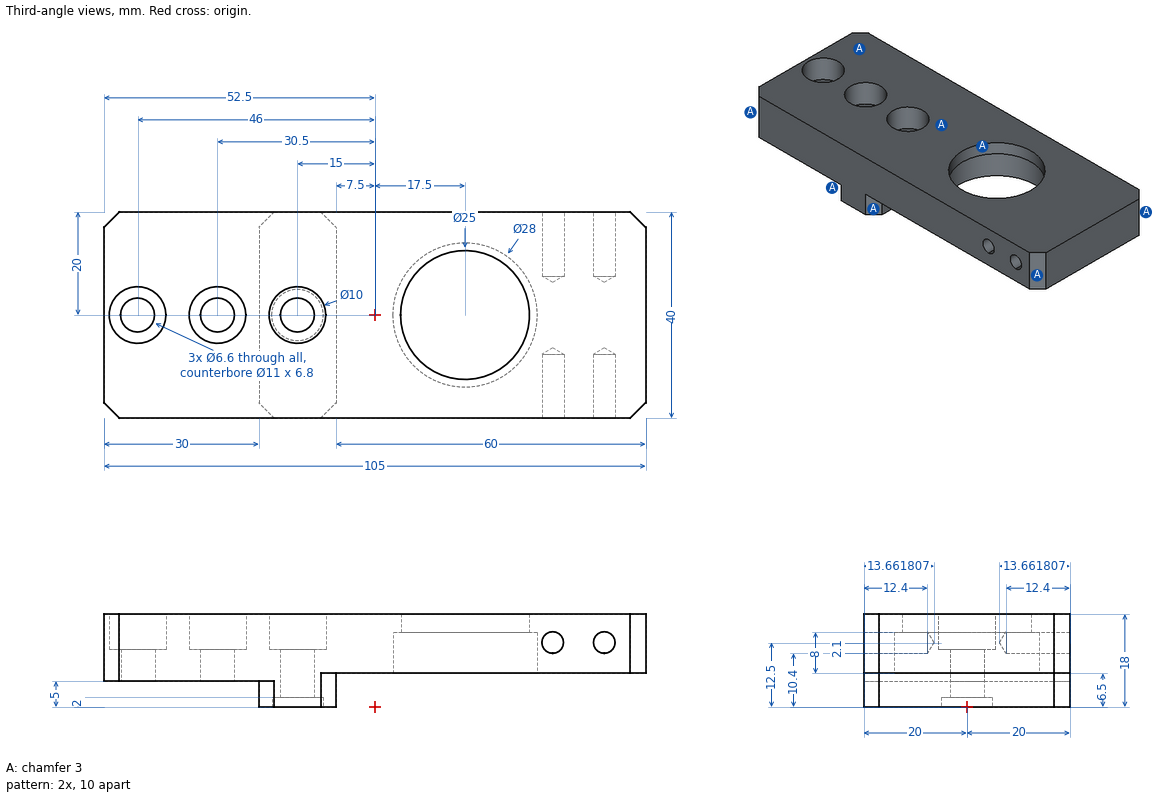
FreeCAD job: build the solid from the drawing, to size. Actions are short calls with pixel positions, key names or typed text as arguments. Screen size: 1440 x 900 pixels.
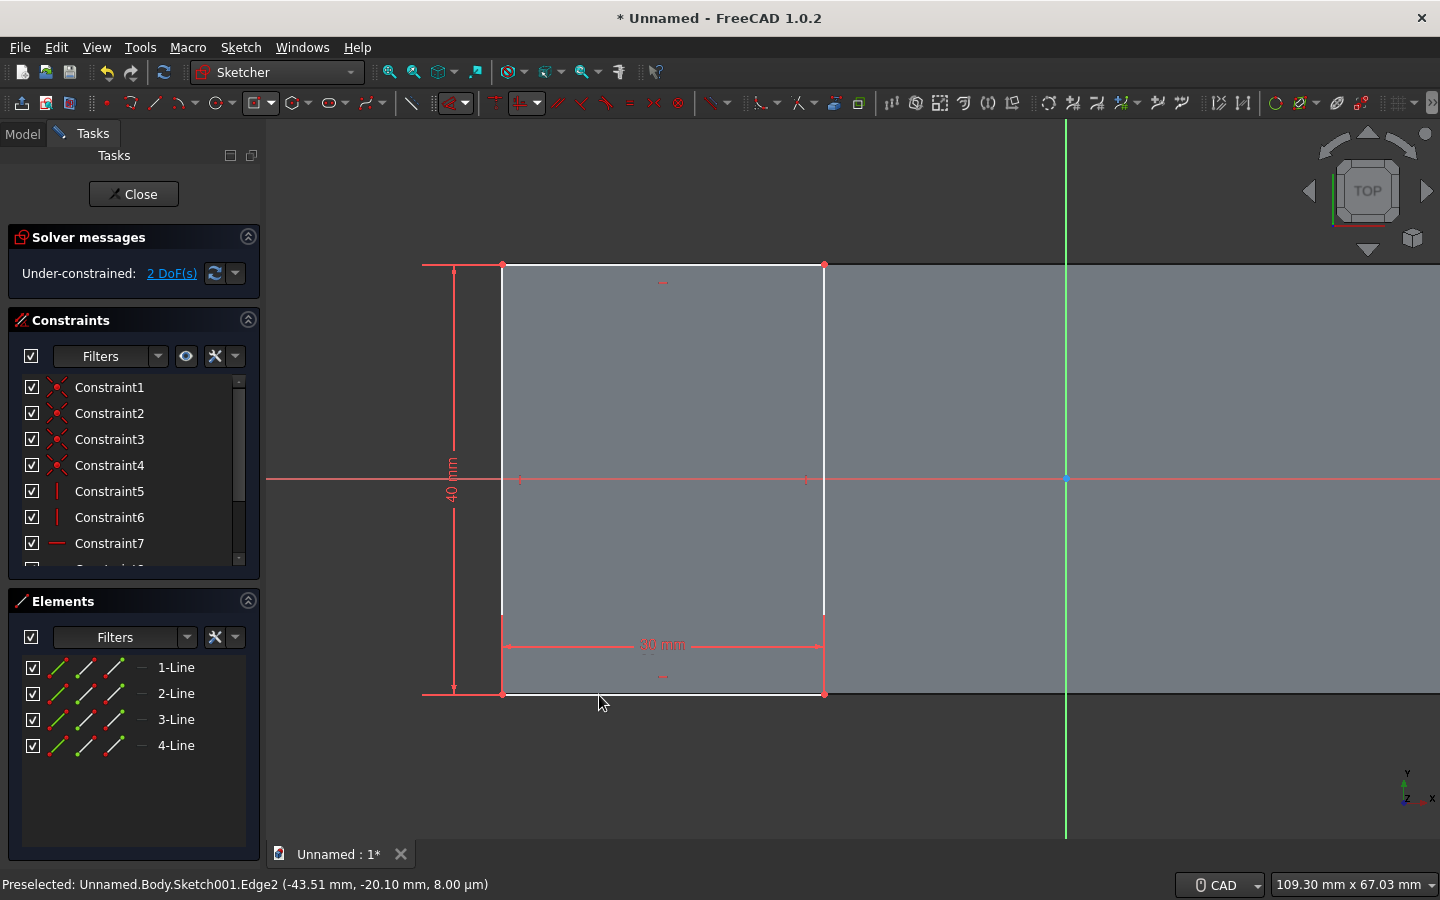
click(502, 265)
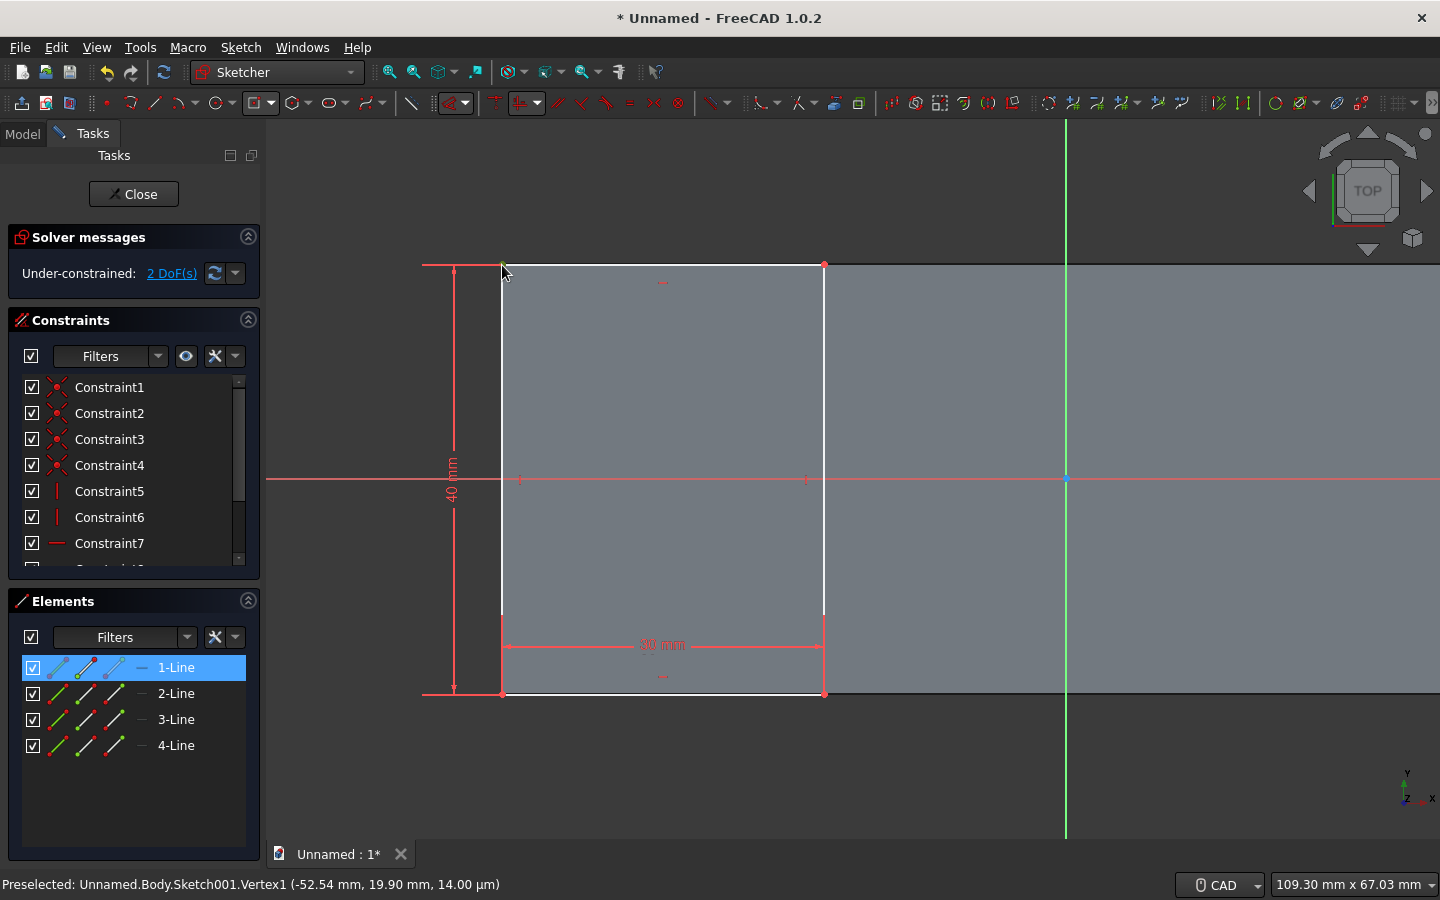
click(468, 104)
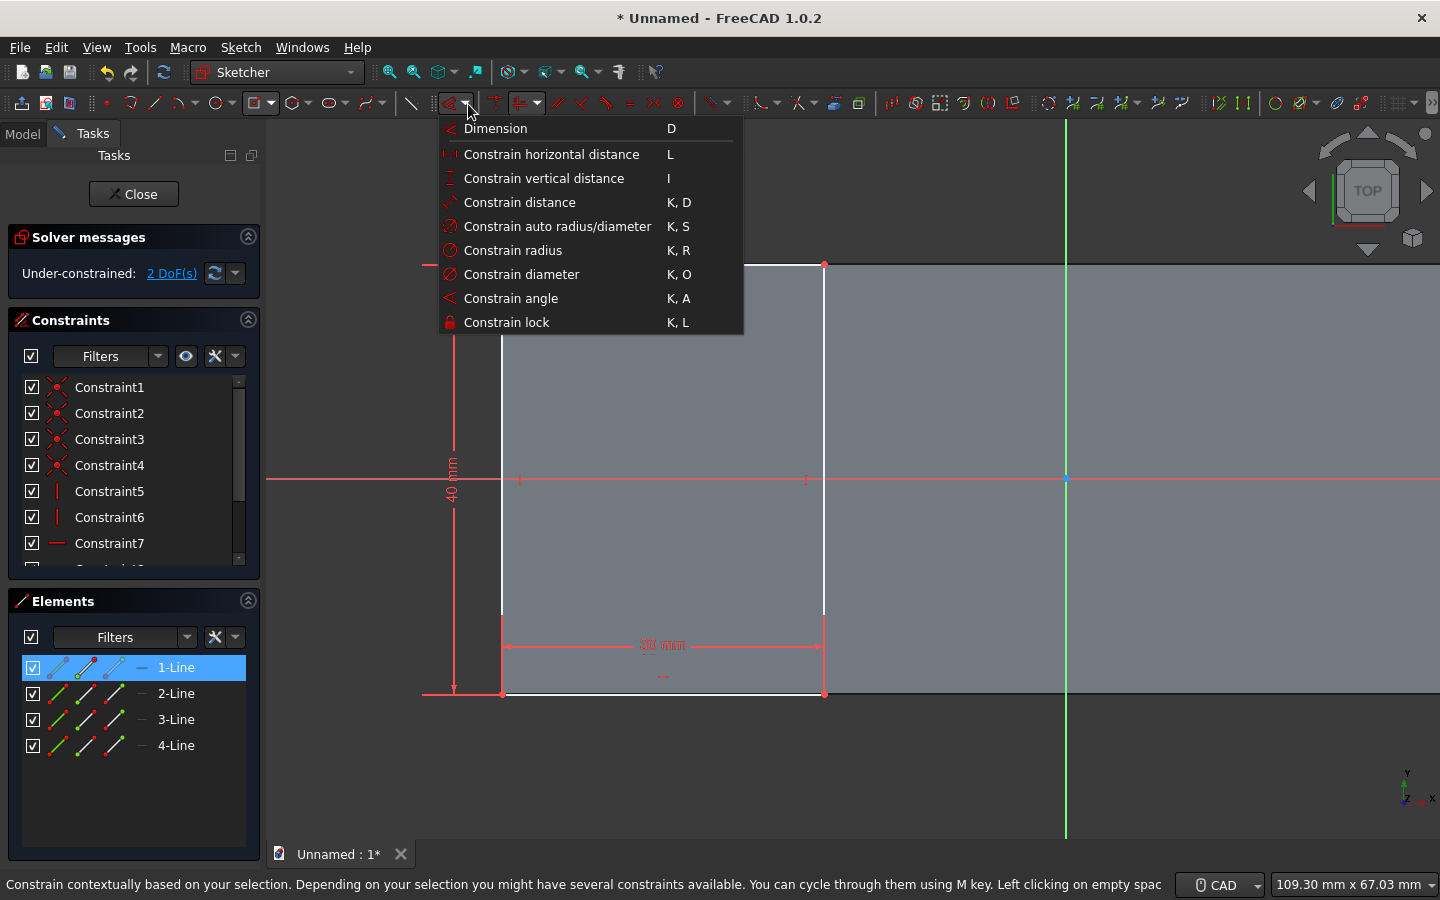
click(591, 178)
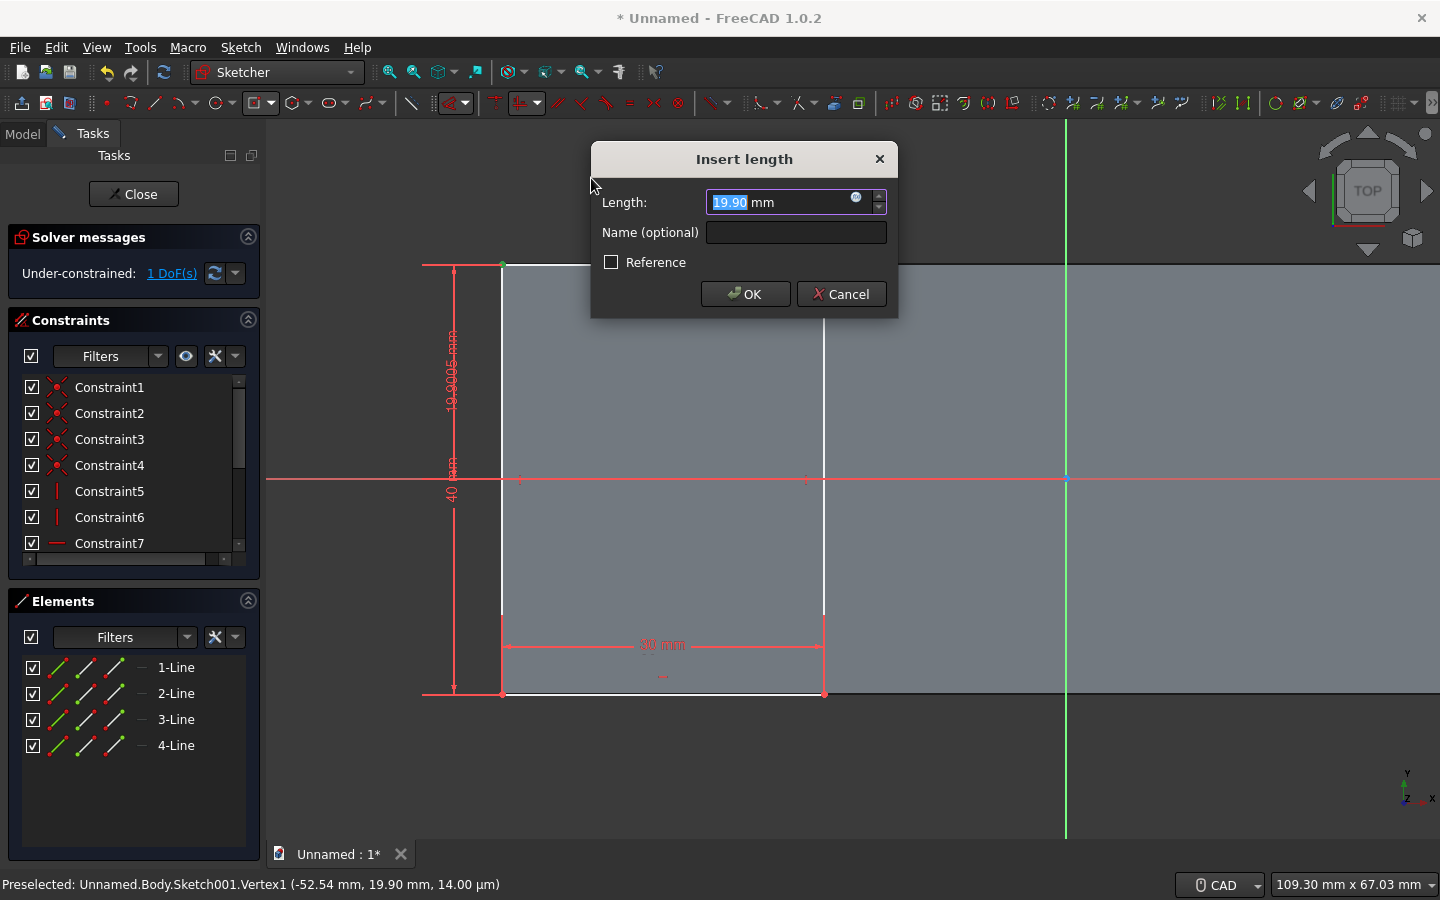
text(20)
key(Return)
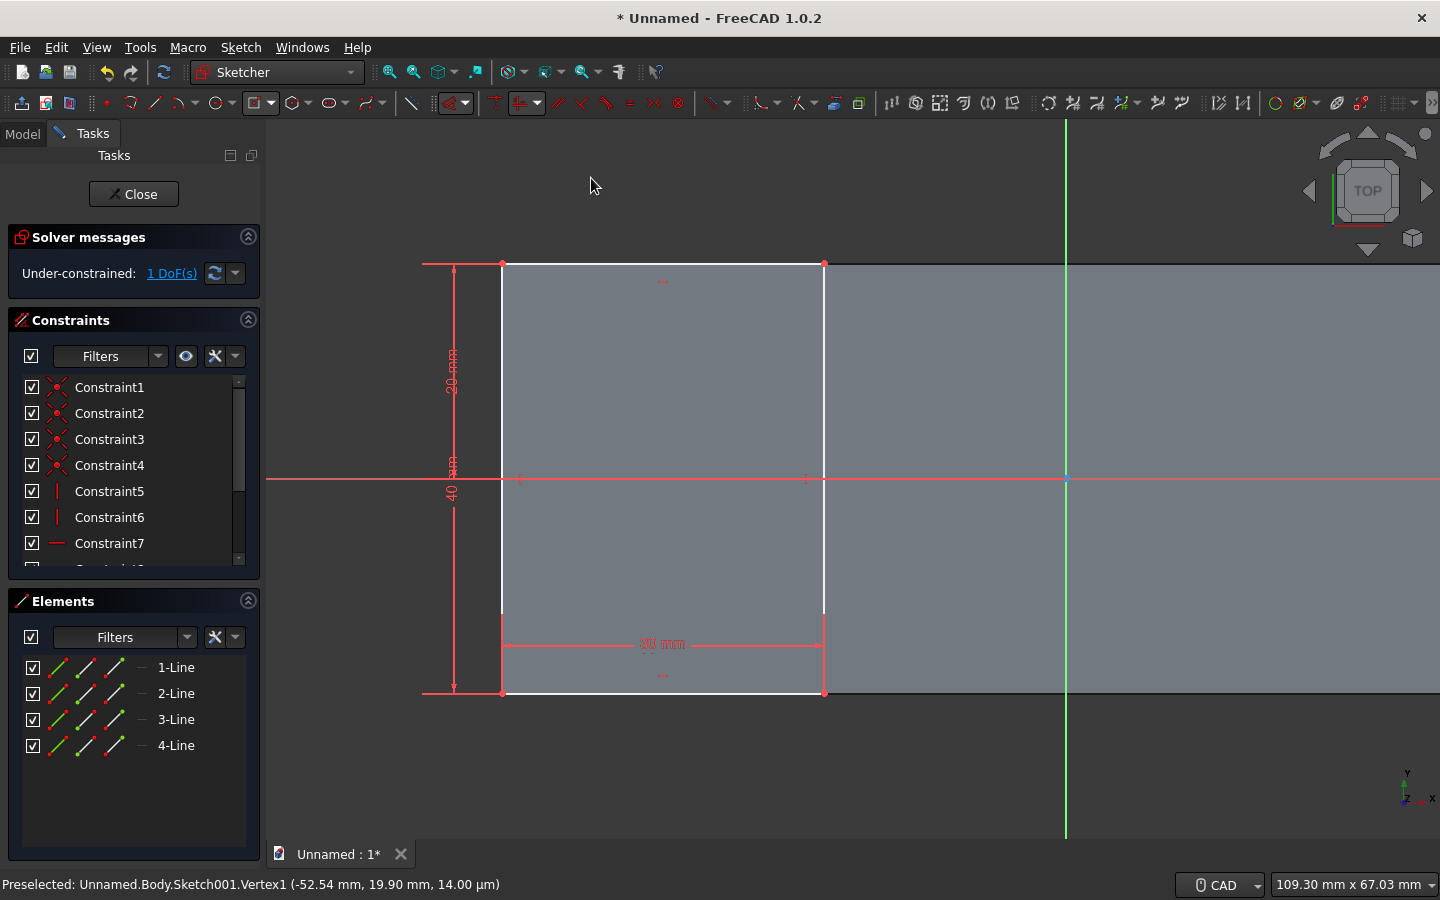
click(502, 264)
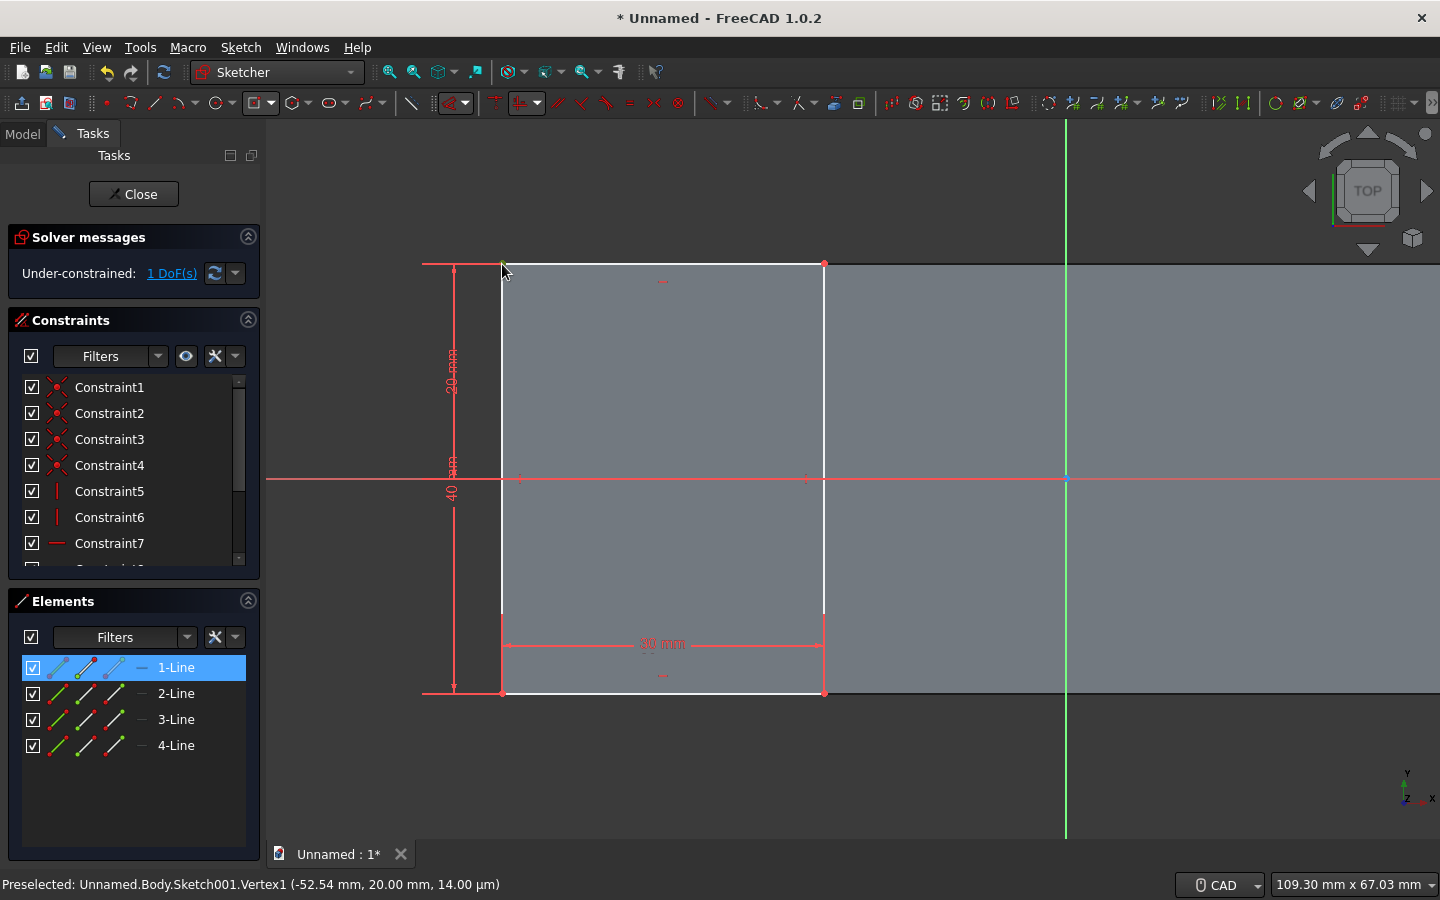
click(468, 104)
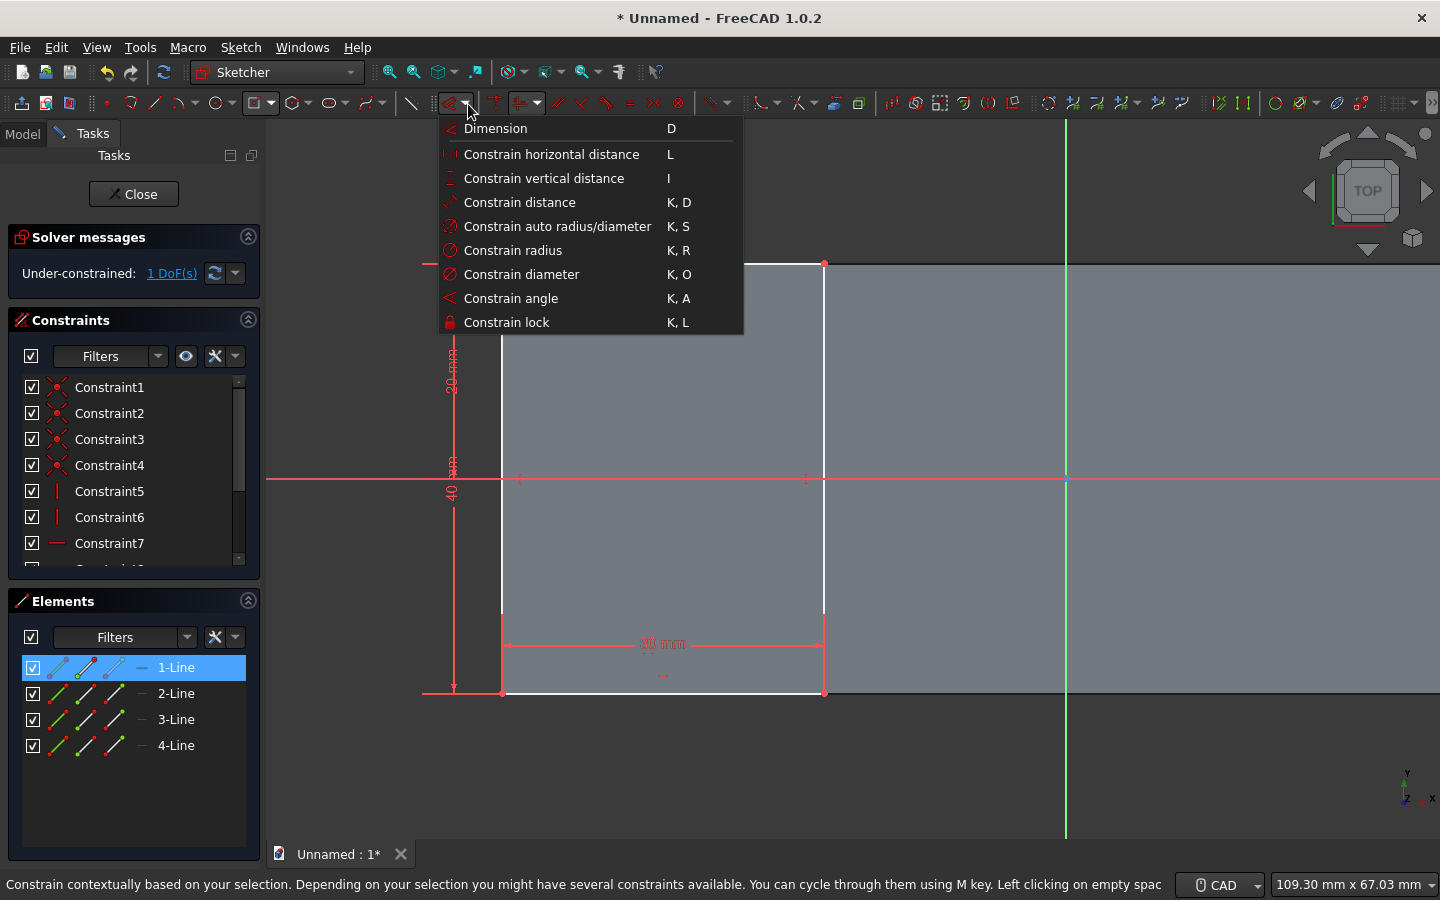
click(591, 154)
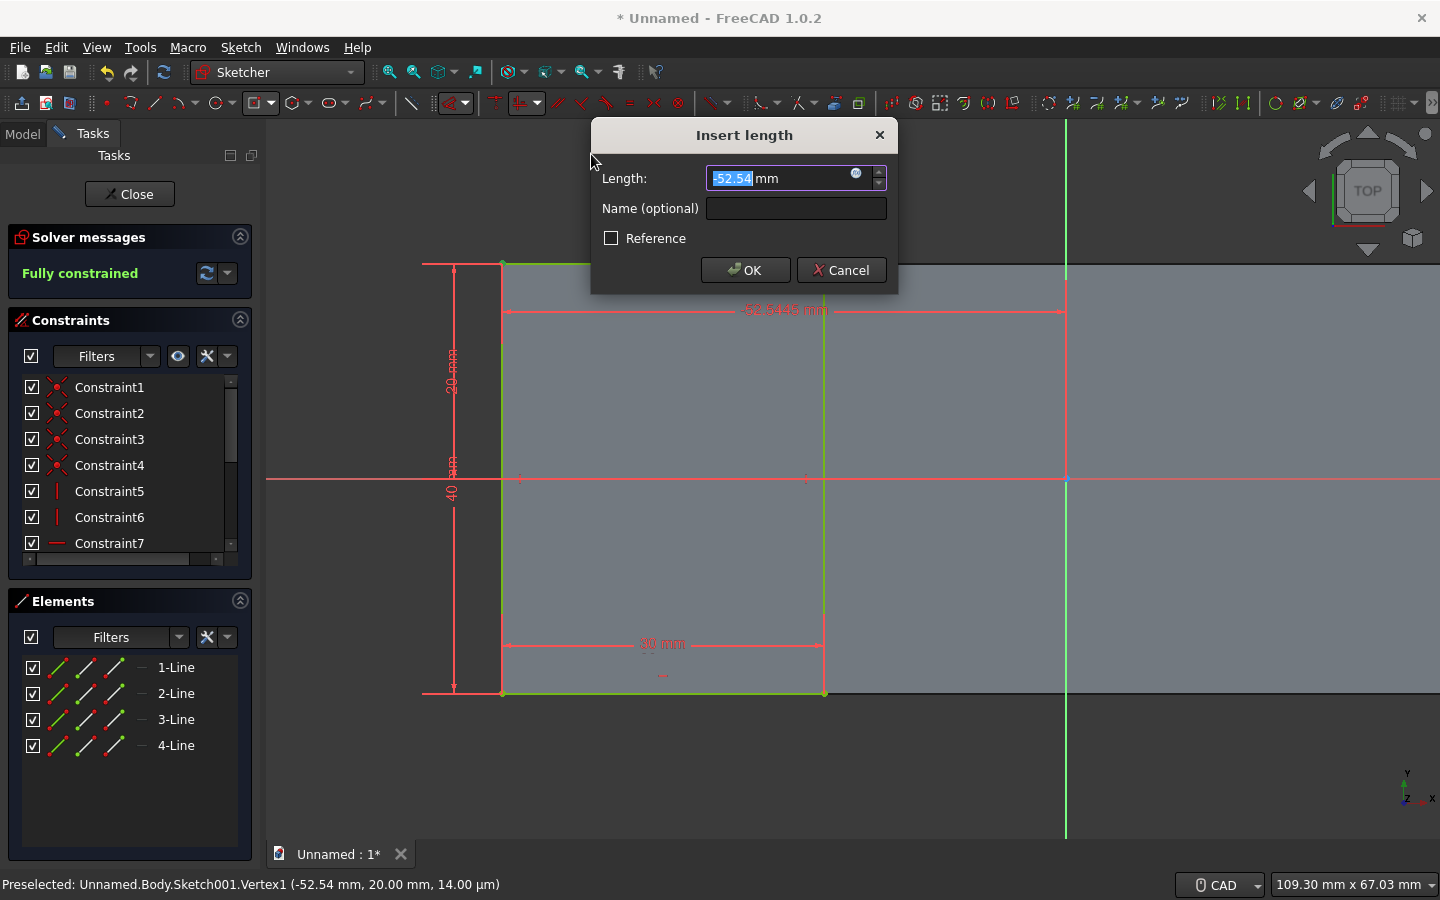
text(-52.5)
key(Return)